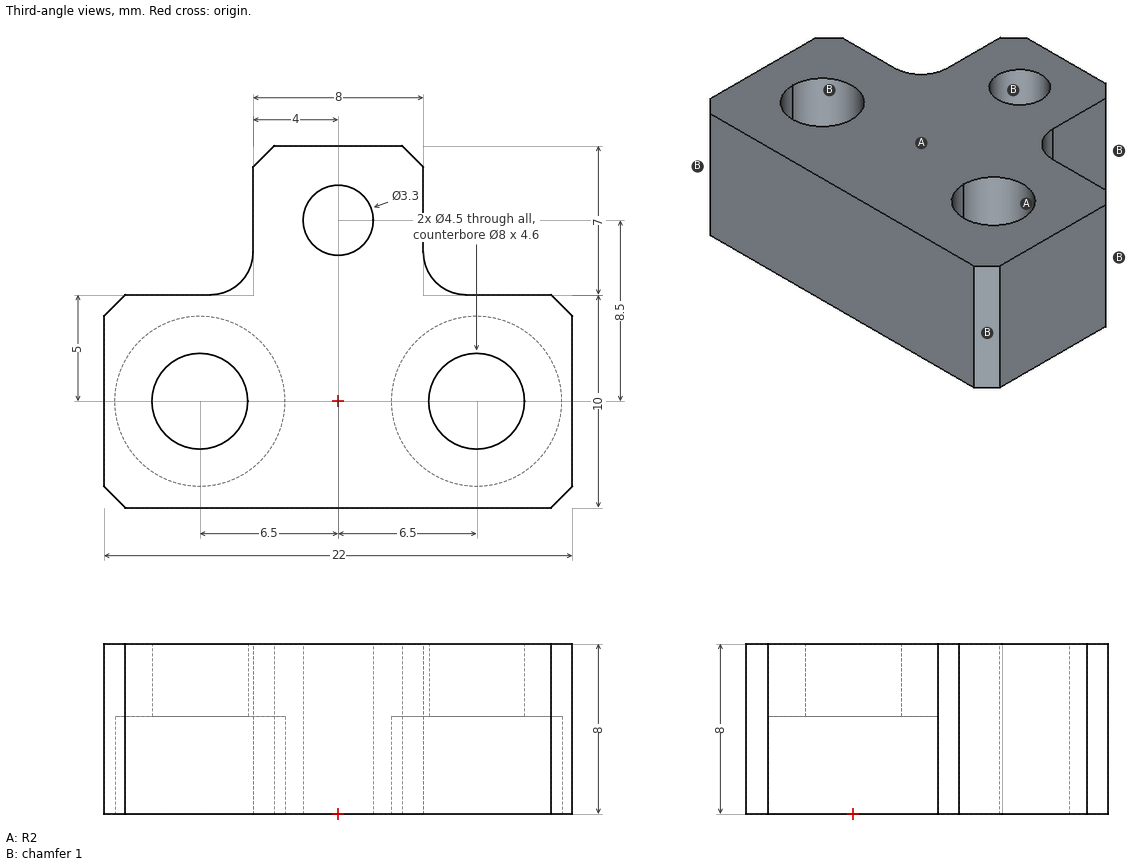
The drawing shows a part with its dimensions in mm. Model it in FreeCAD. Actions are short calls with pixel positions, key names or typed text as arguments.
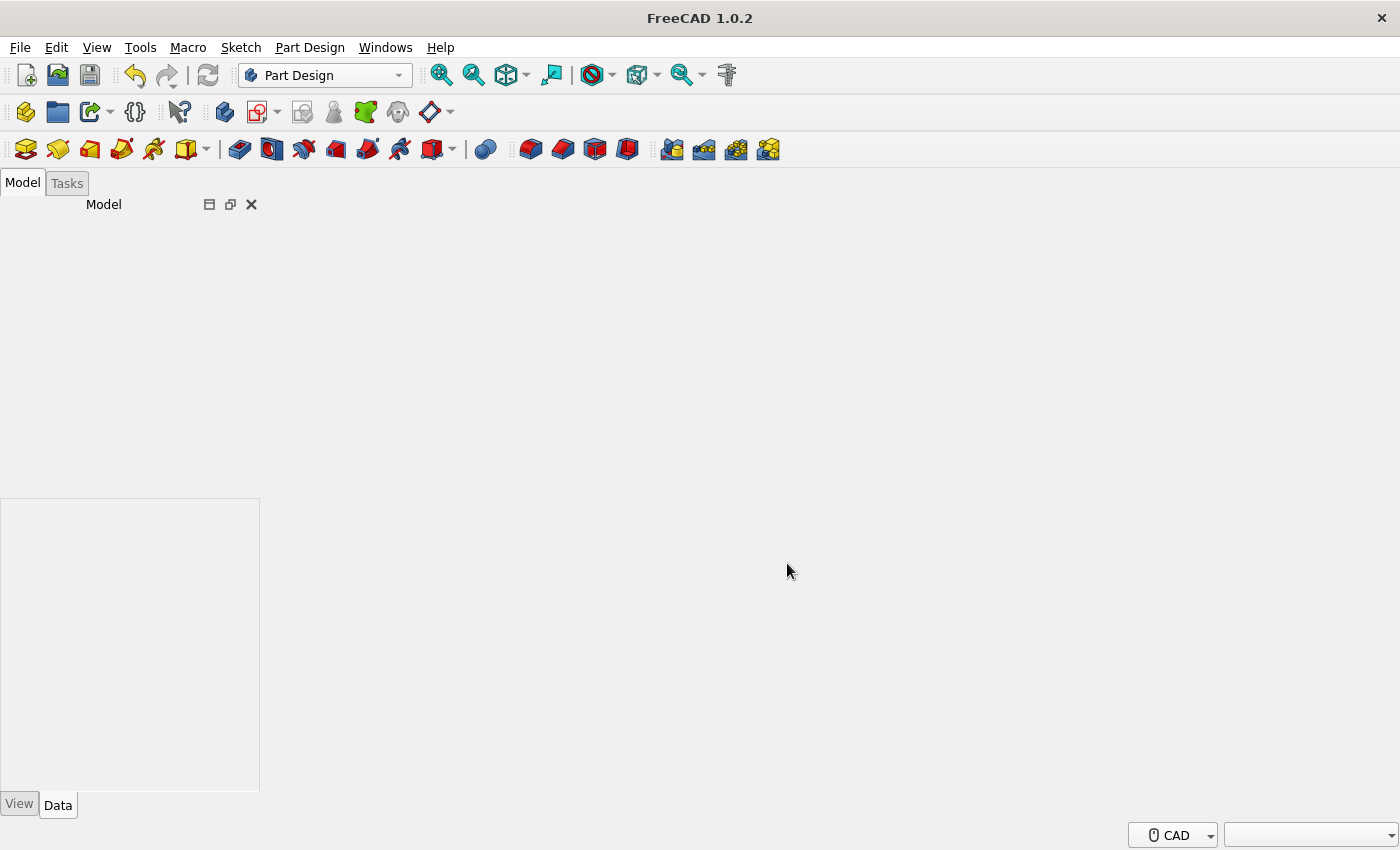
click(26, 76)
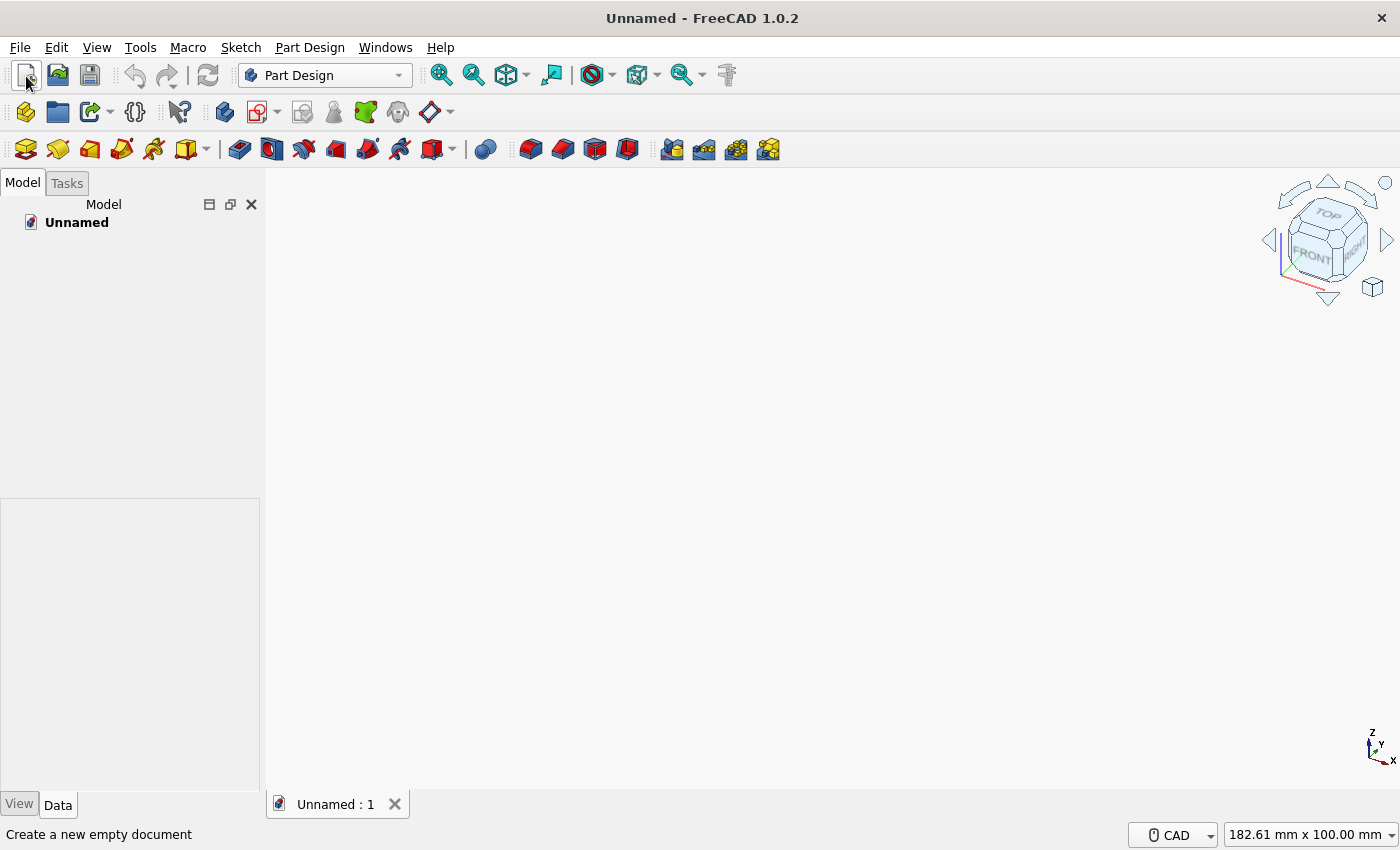
click(258, 112)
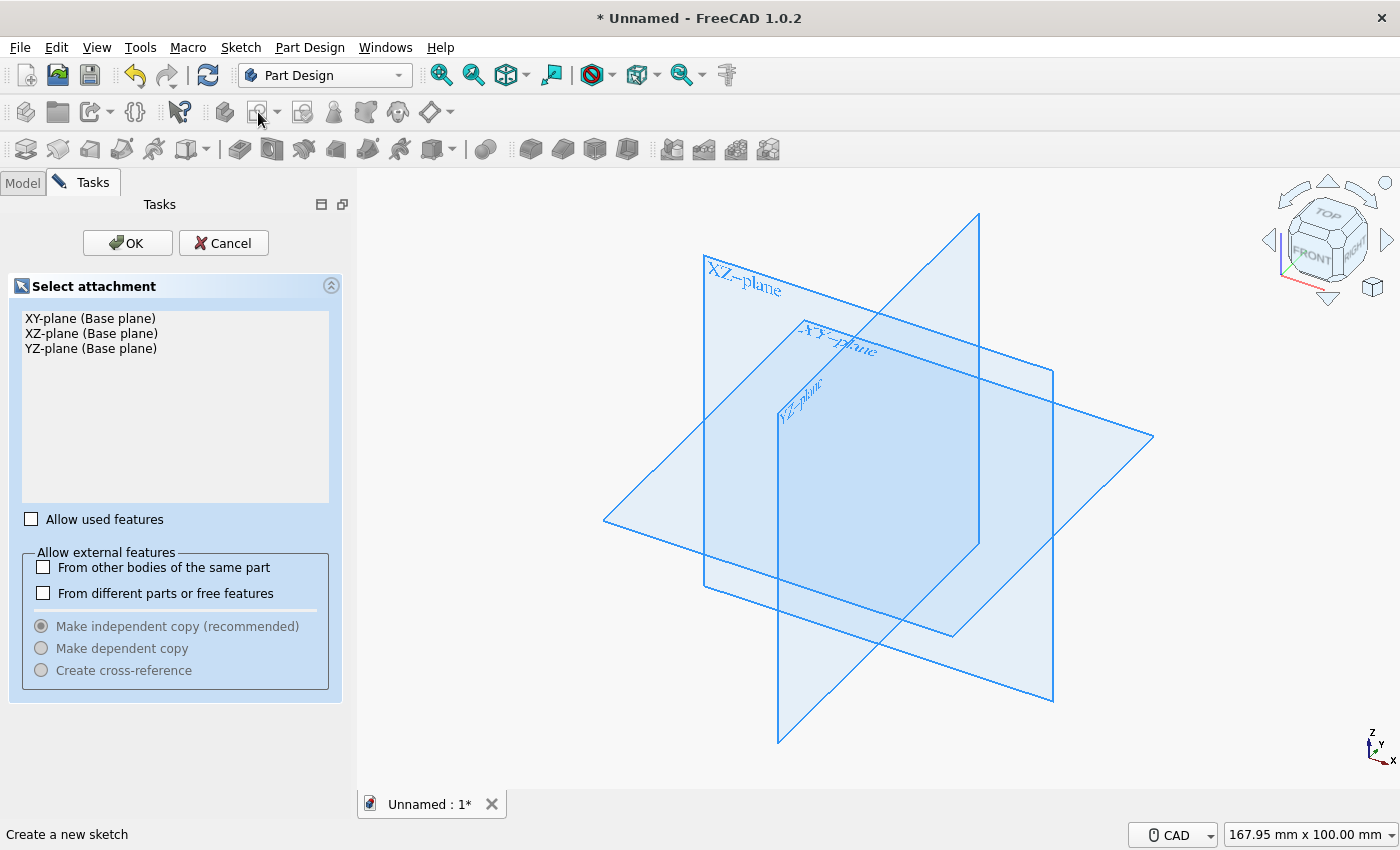
click(82, 318)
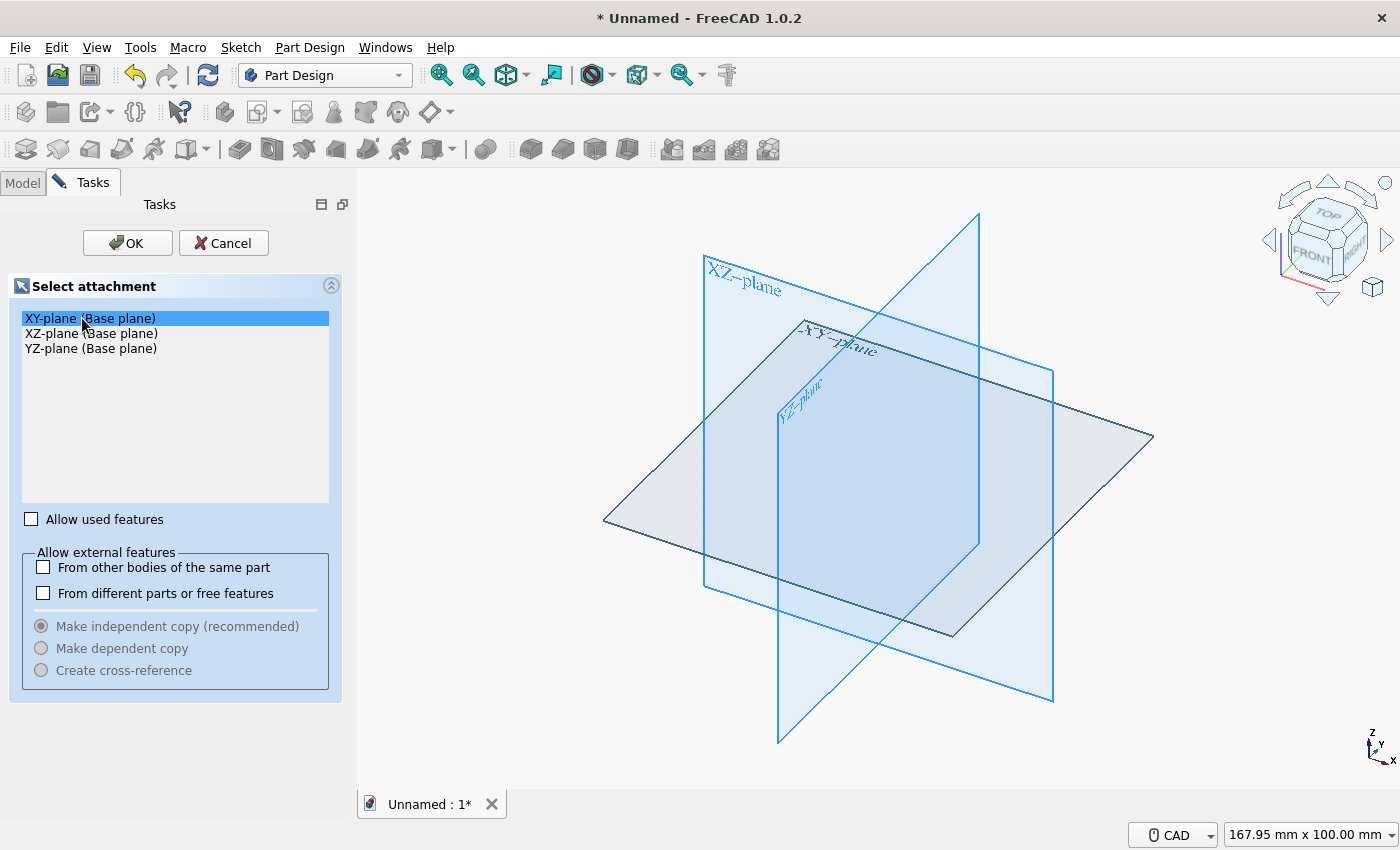
click(128, 243)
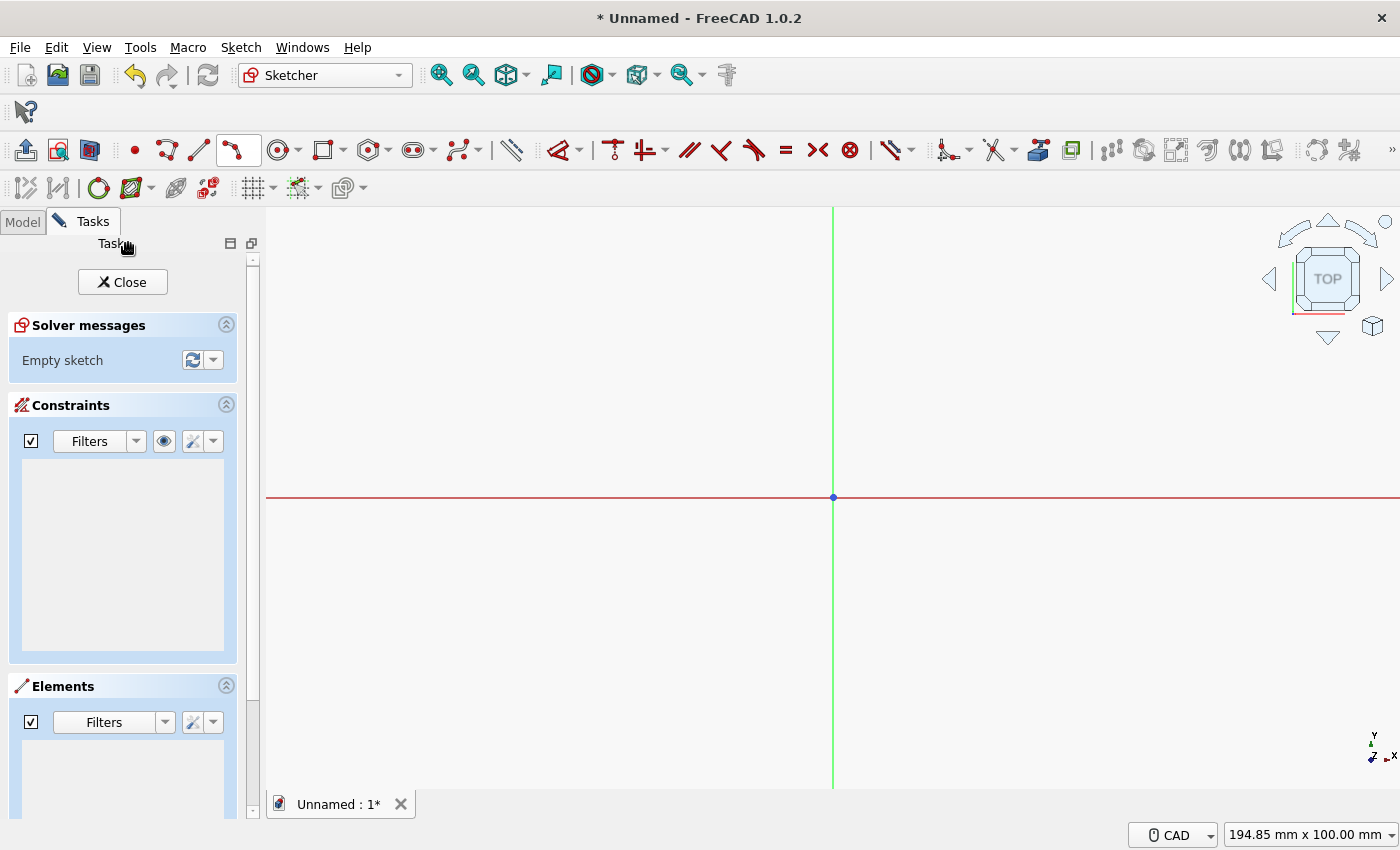
scroll(850, 498, up, 8)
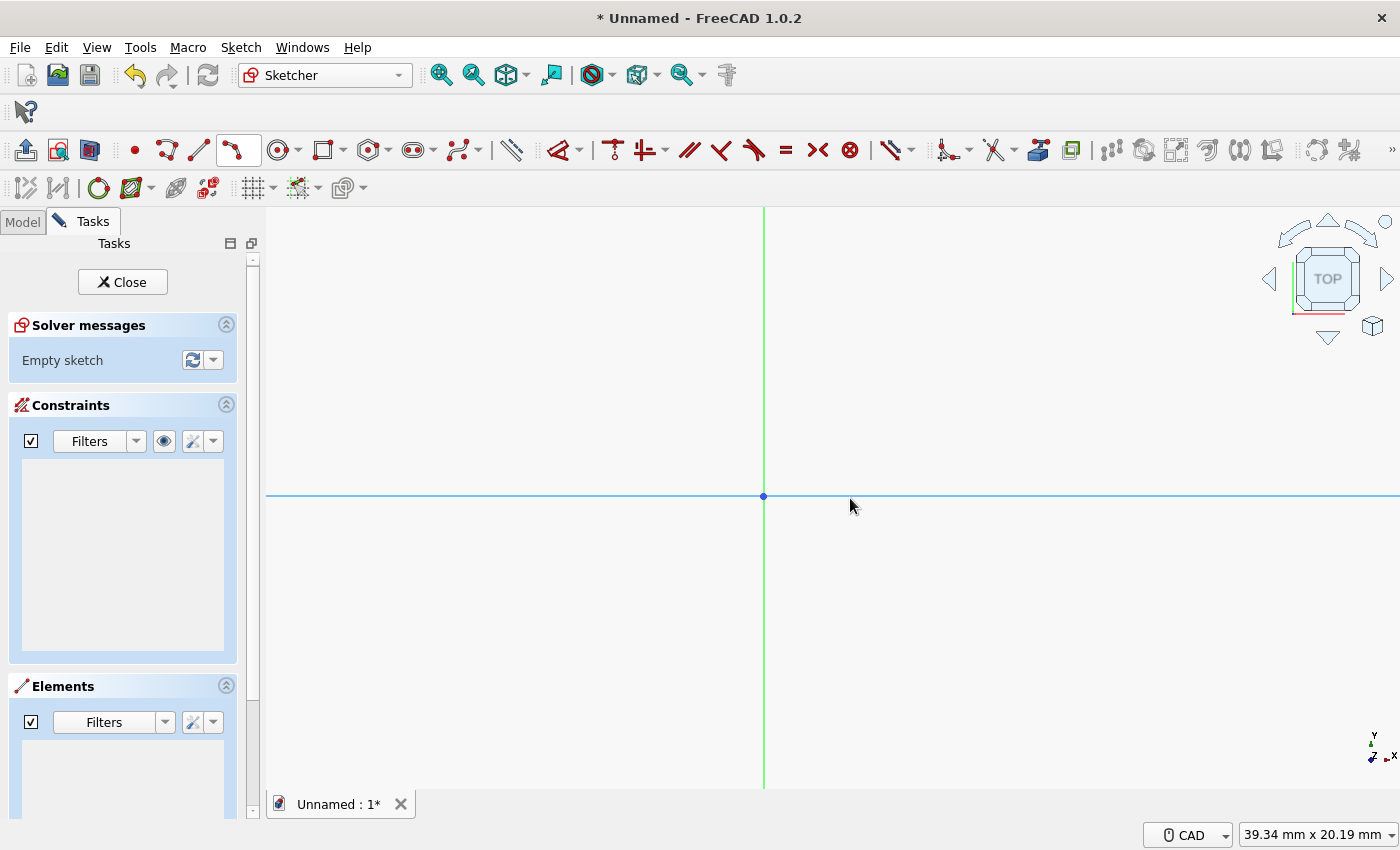
key(g)
key(v)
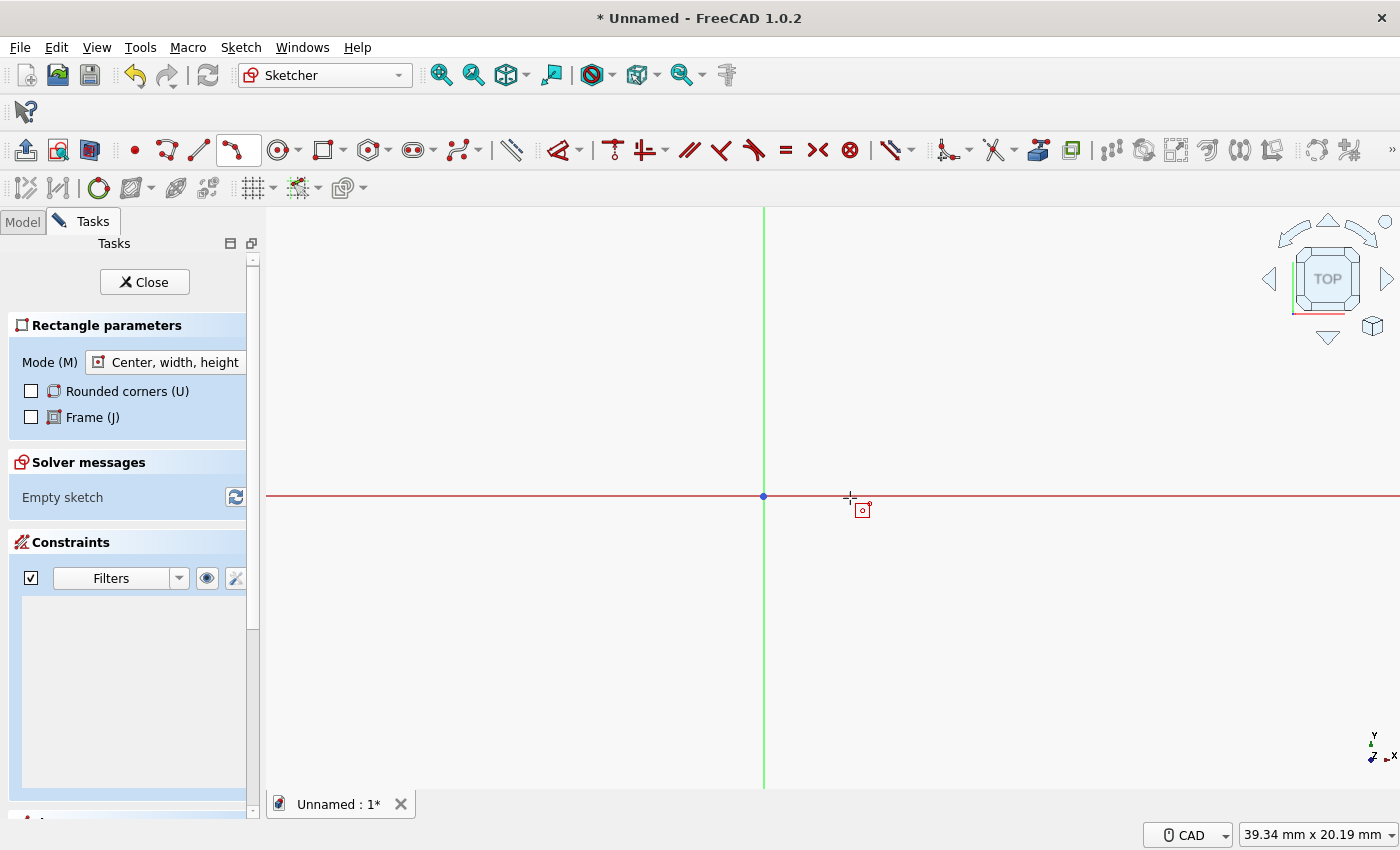
click(764, 496)
move(1081, 352)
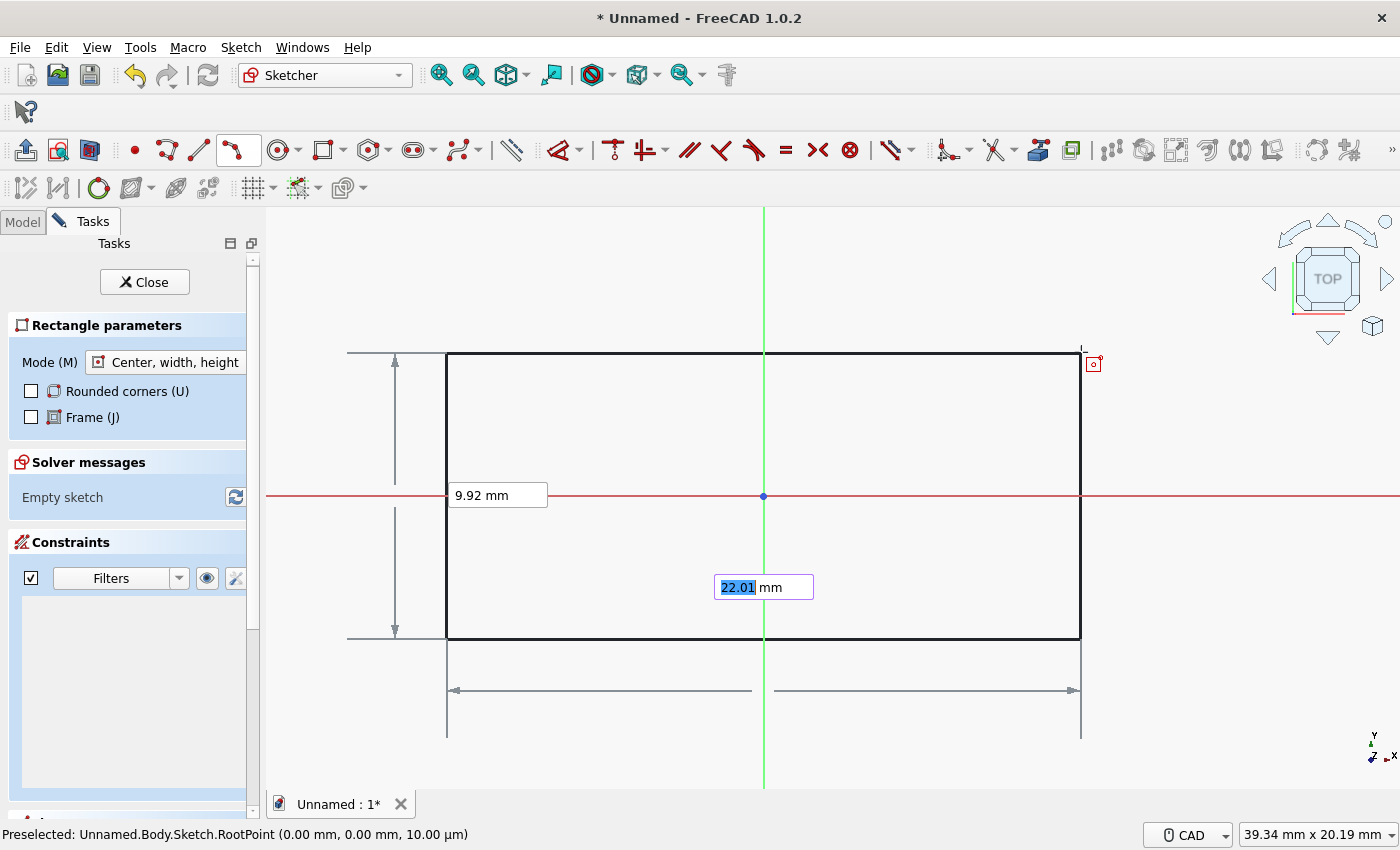
text(22)
key(Tab)
text(10)
key(Return)
key(Escape)